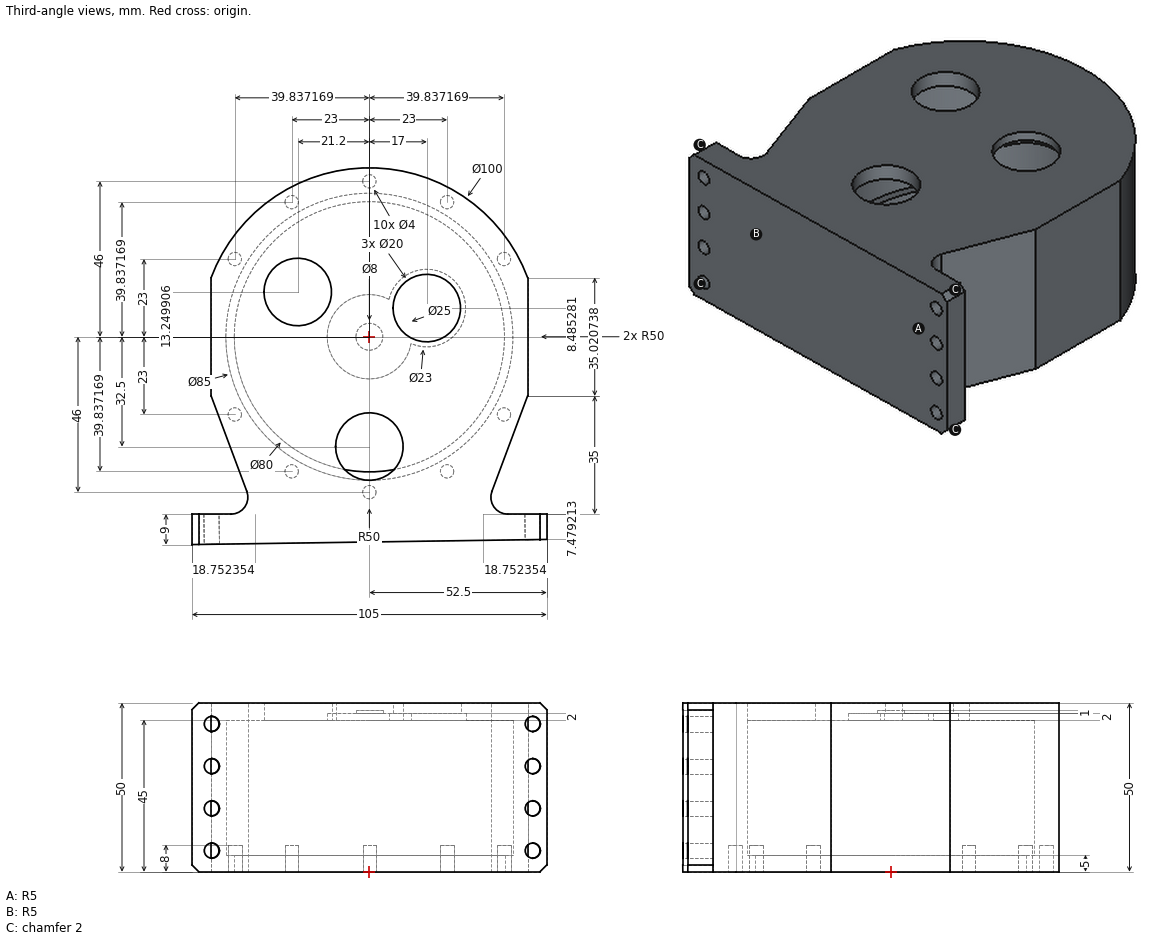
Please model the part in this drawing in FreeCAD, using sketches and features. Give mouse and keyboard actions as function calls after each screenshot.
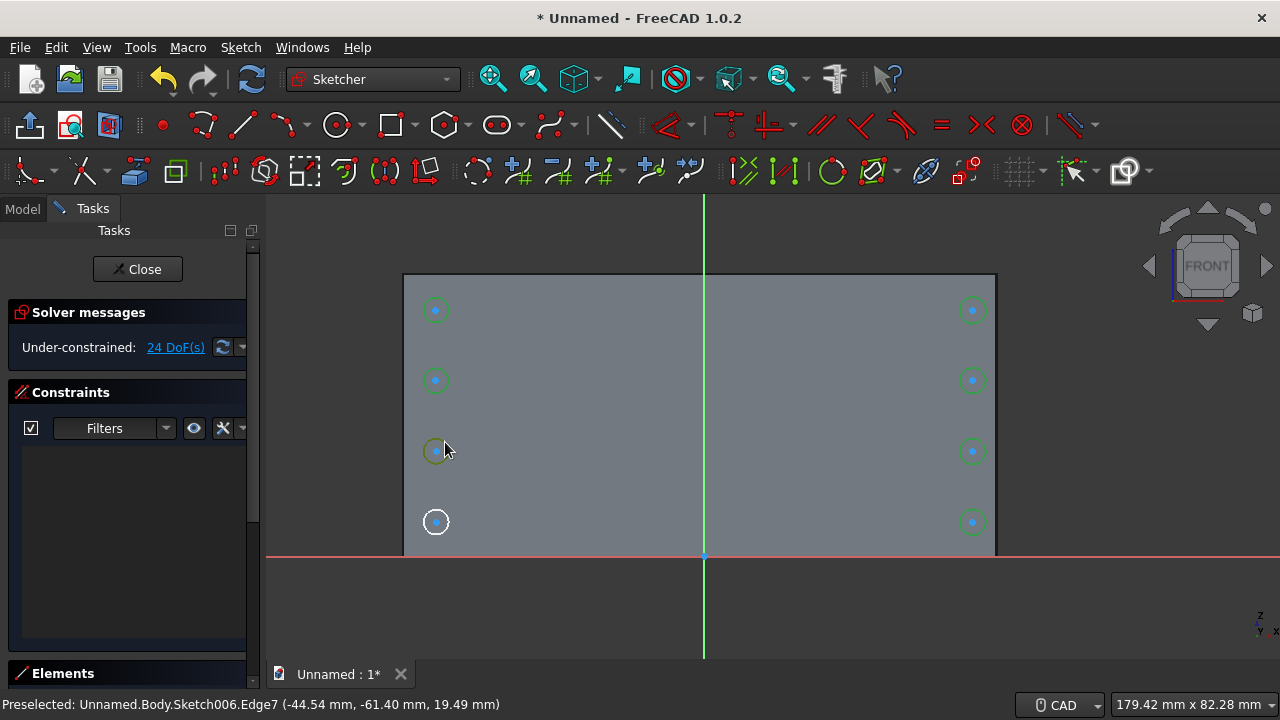
click(445, 513)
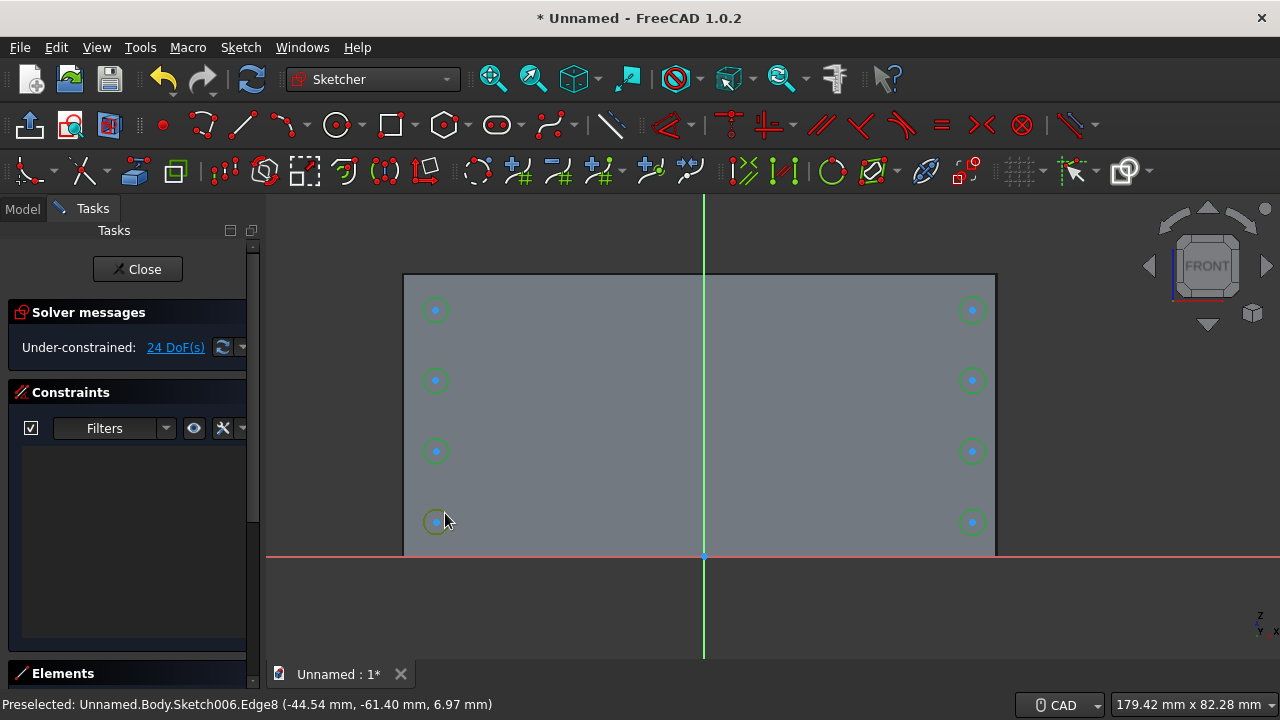
key(e)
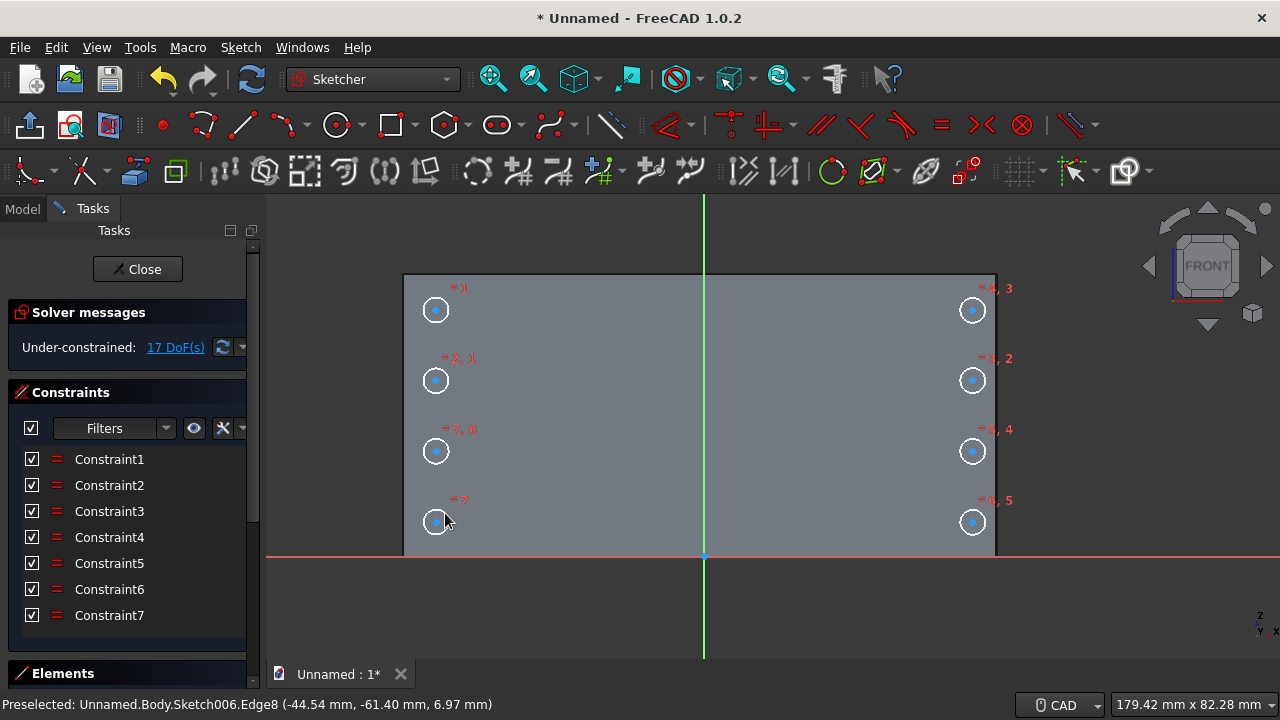
click(436, 310)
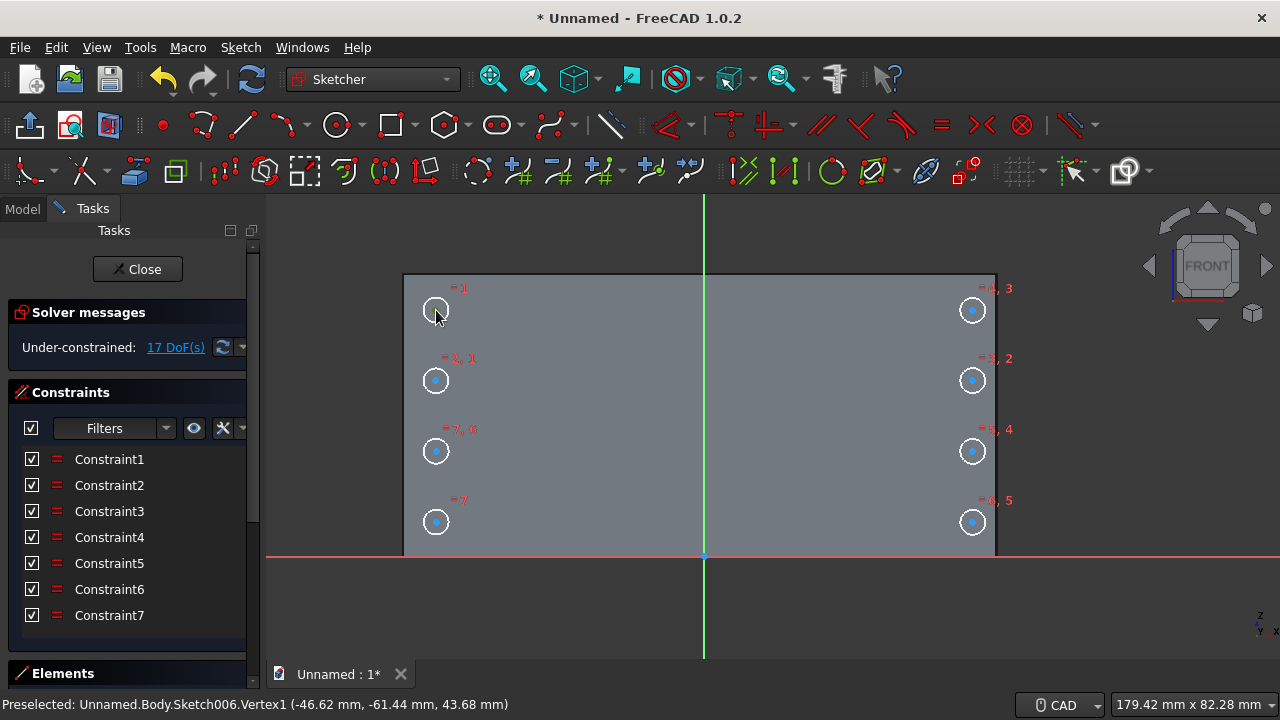
click(436, 381)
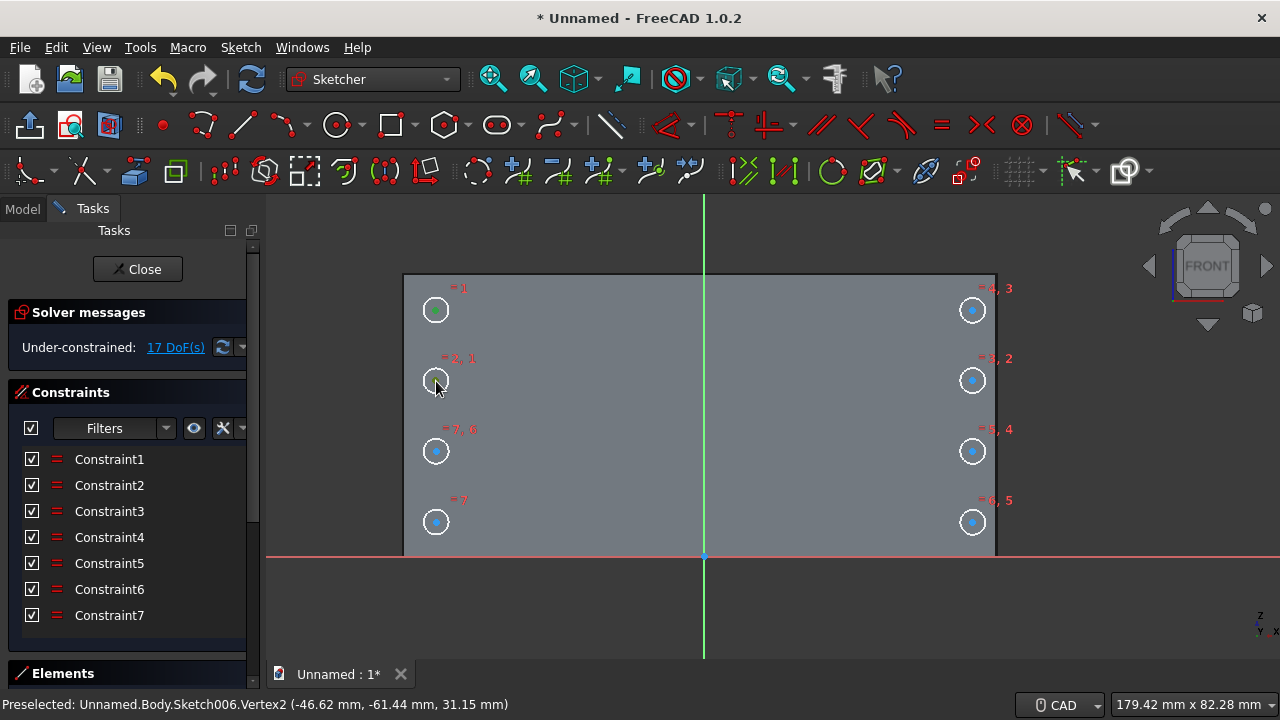
key(v)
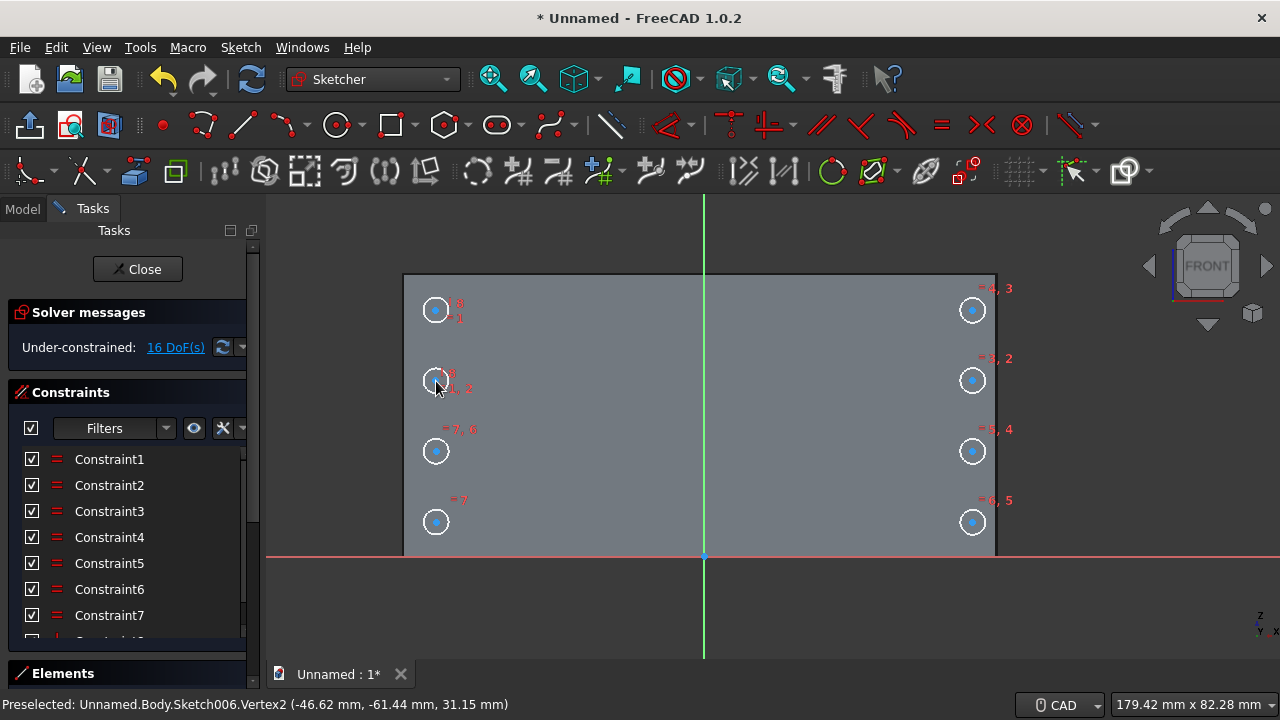
click(436, 381)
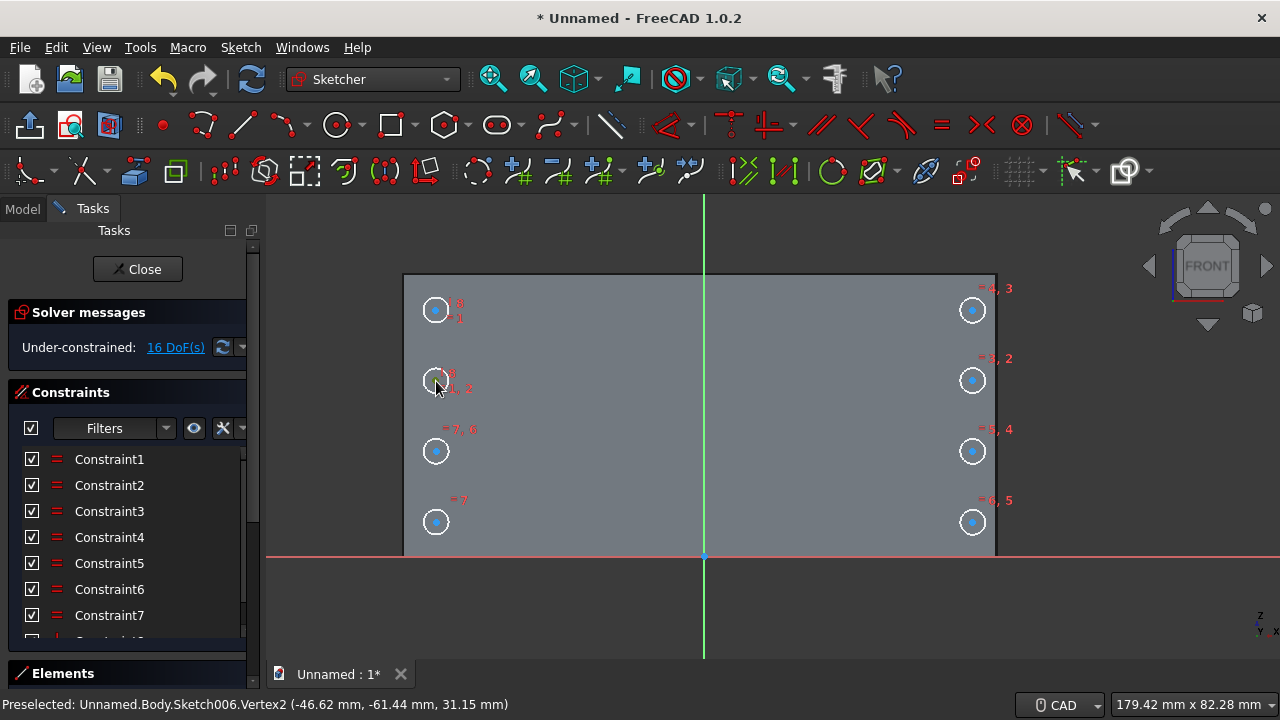
click(973, 381)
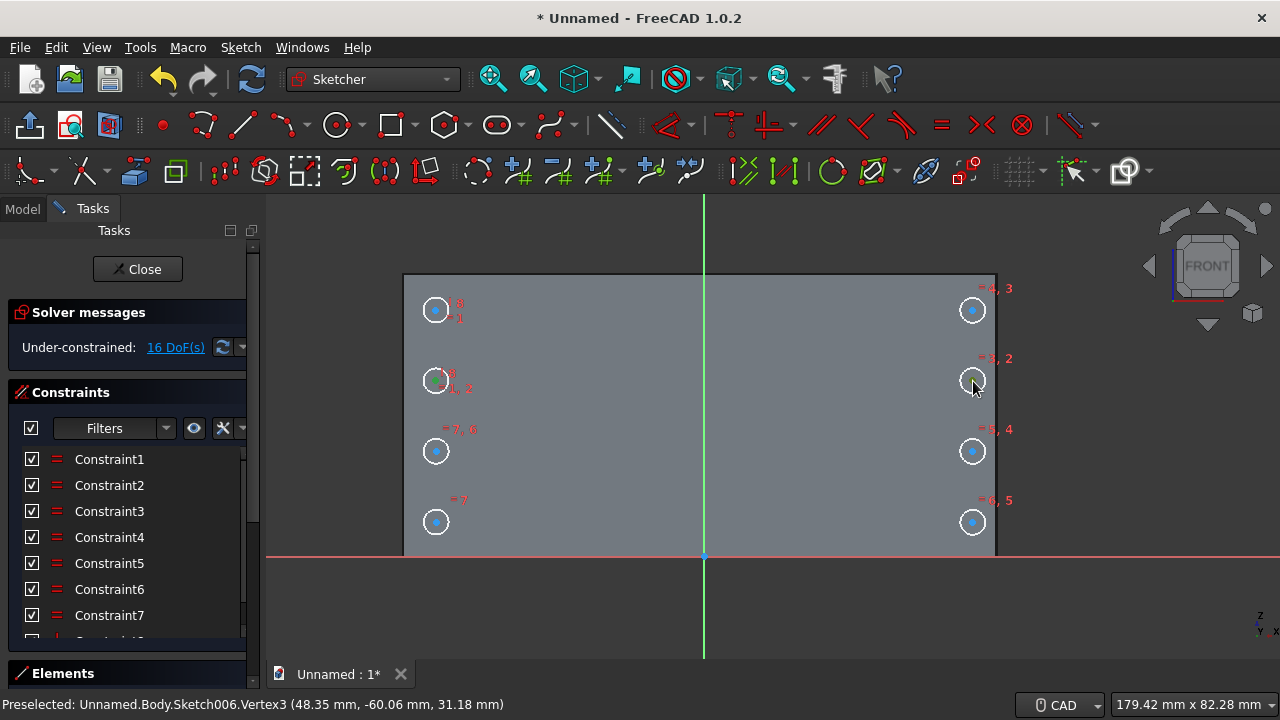
click(796, 126)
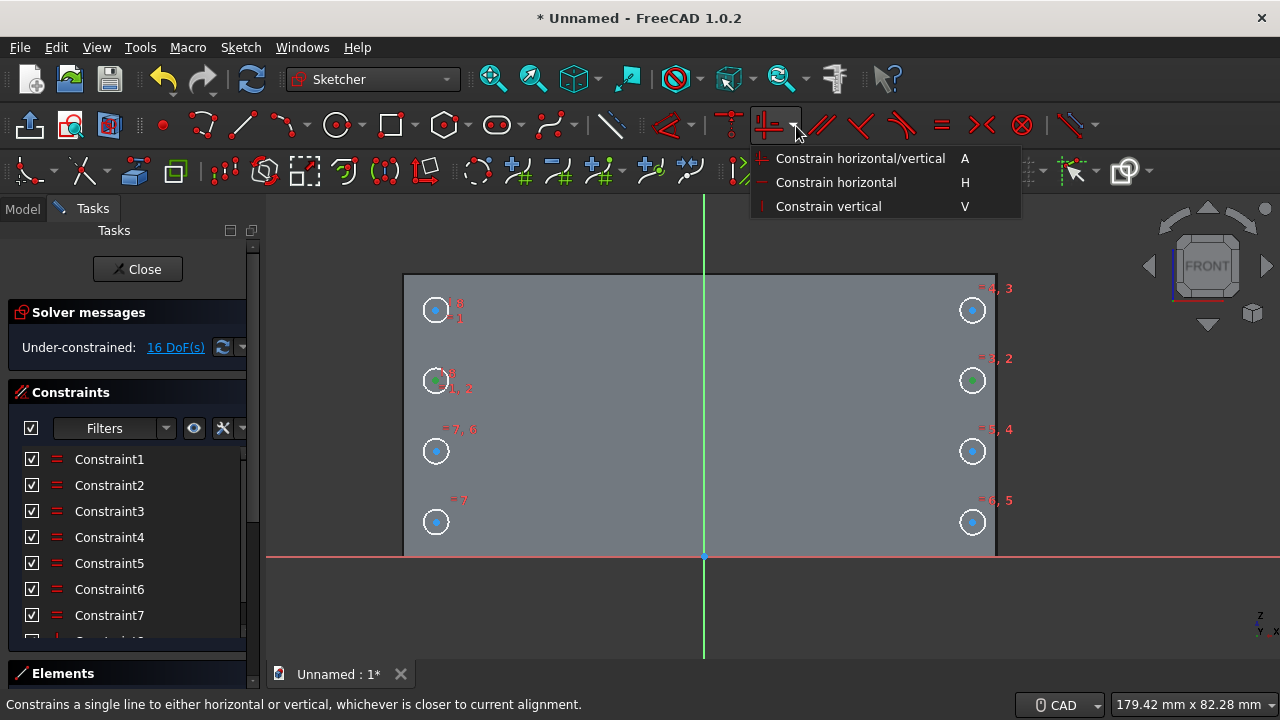
click(886, 182)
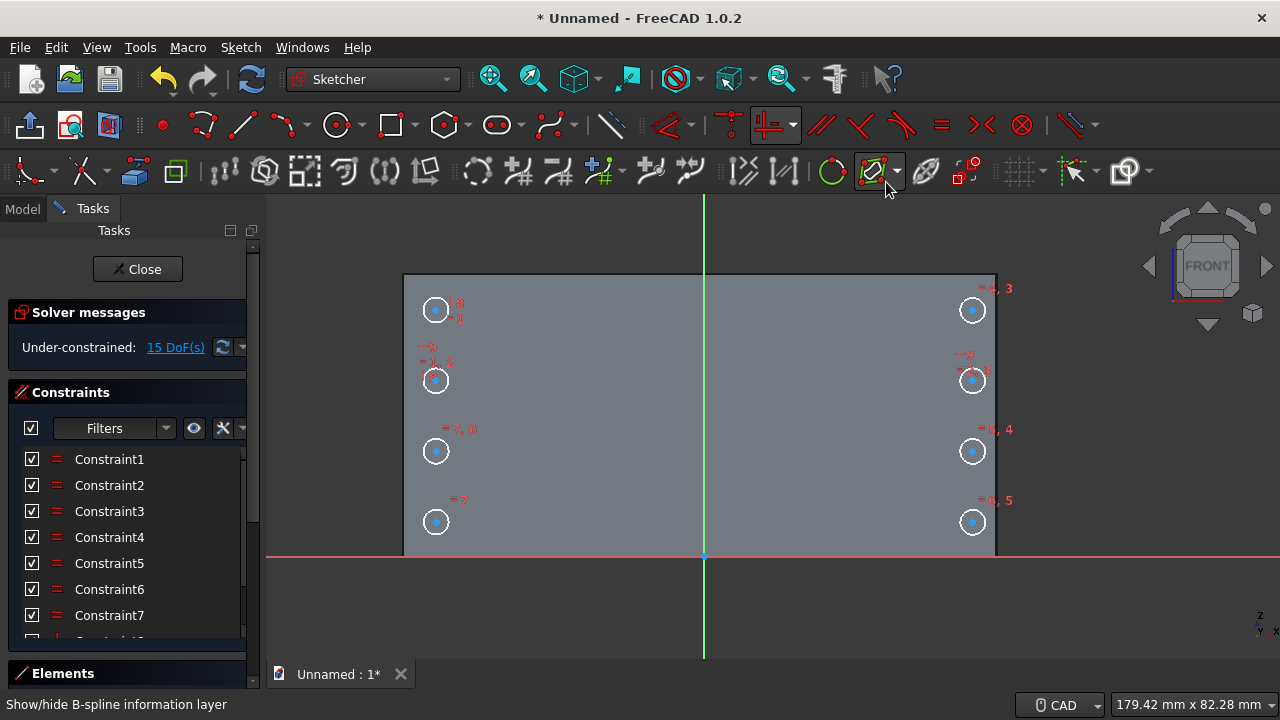
click(973, 381)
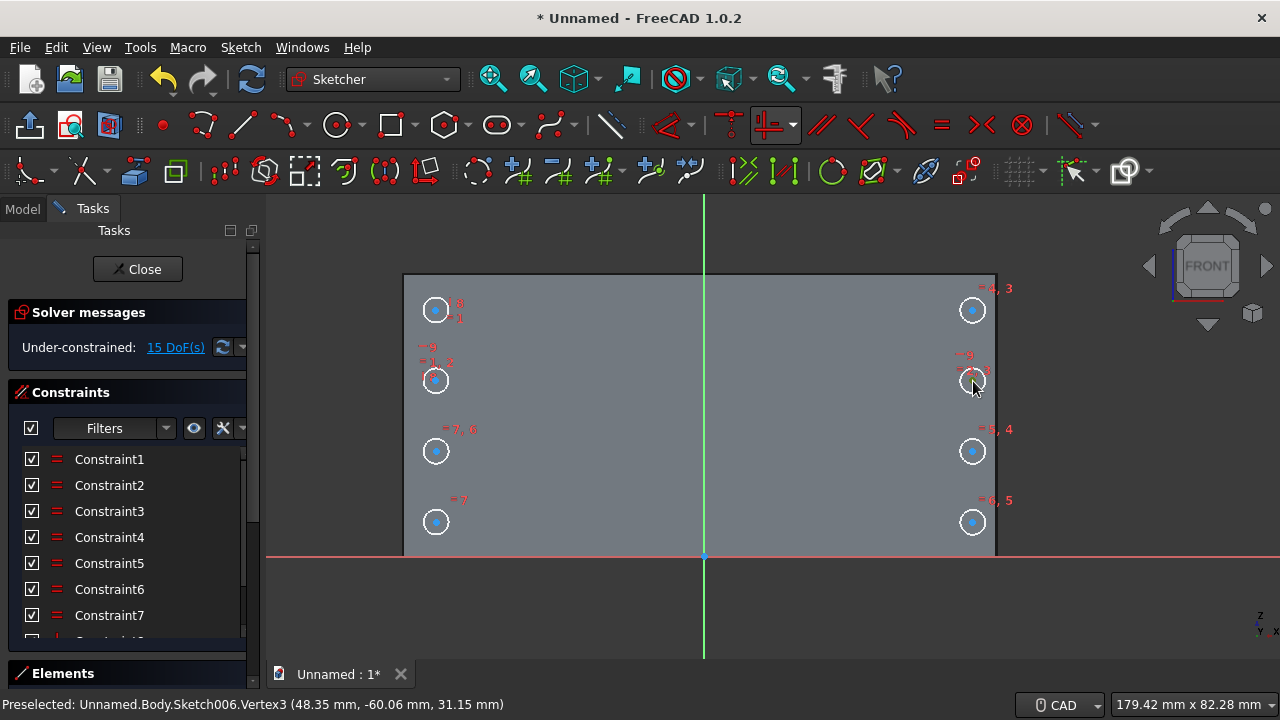
click(973, 310)